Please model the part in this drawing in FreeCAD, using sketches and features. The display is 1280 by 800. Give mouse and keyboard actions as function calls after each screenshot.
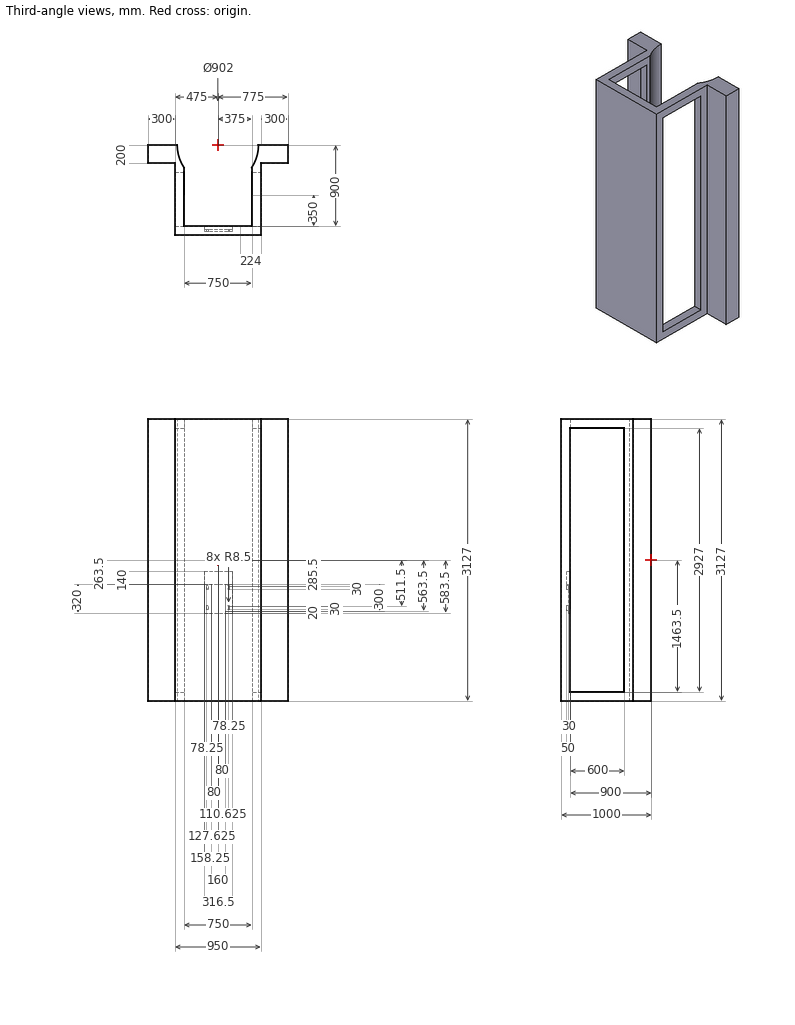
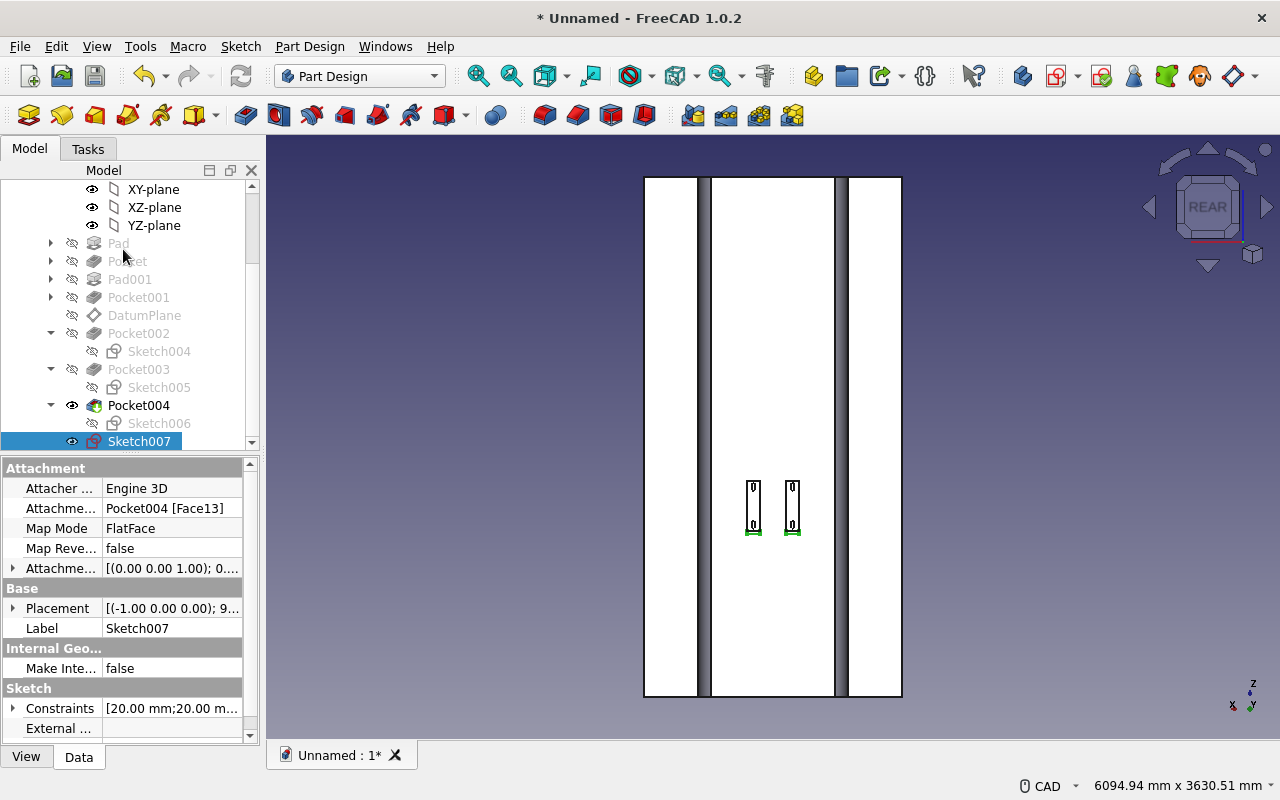
click(246, 116)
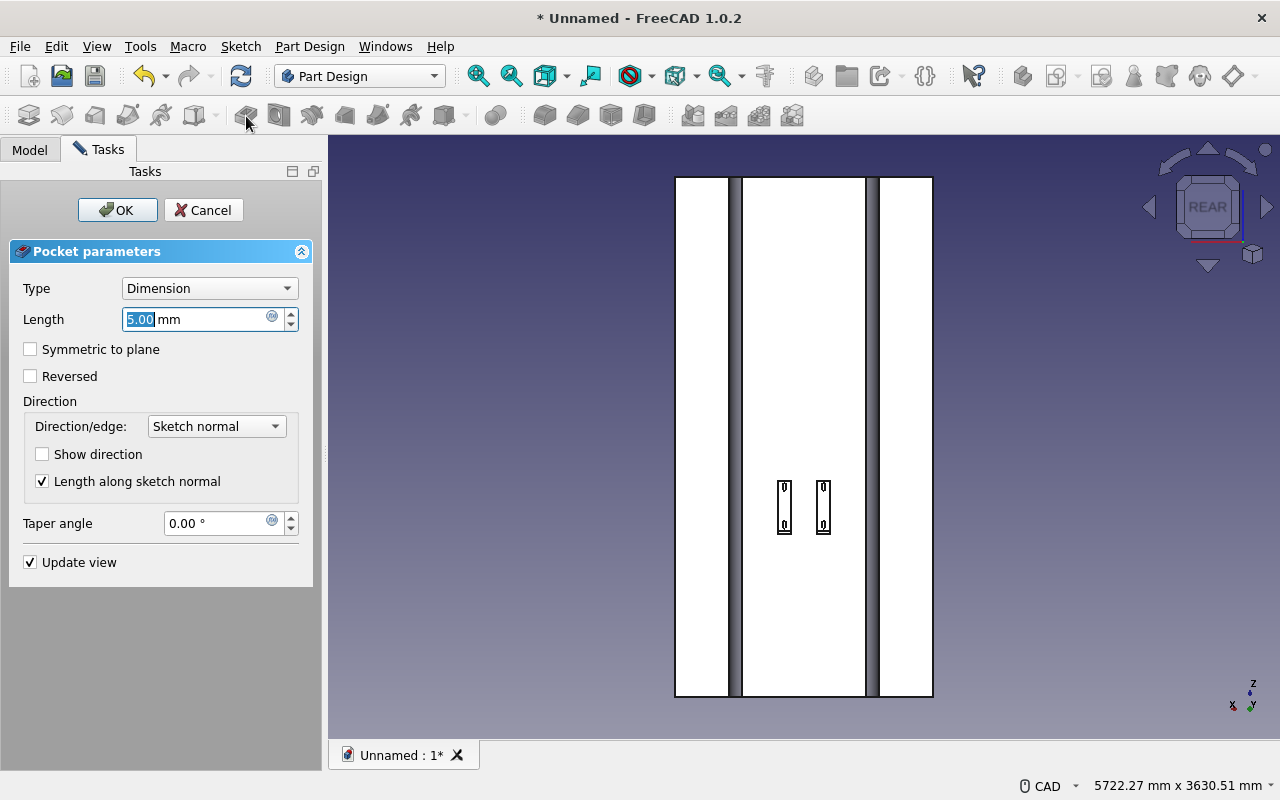
text(30)
key(Tab)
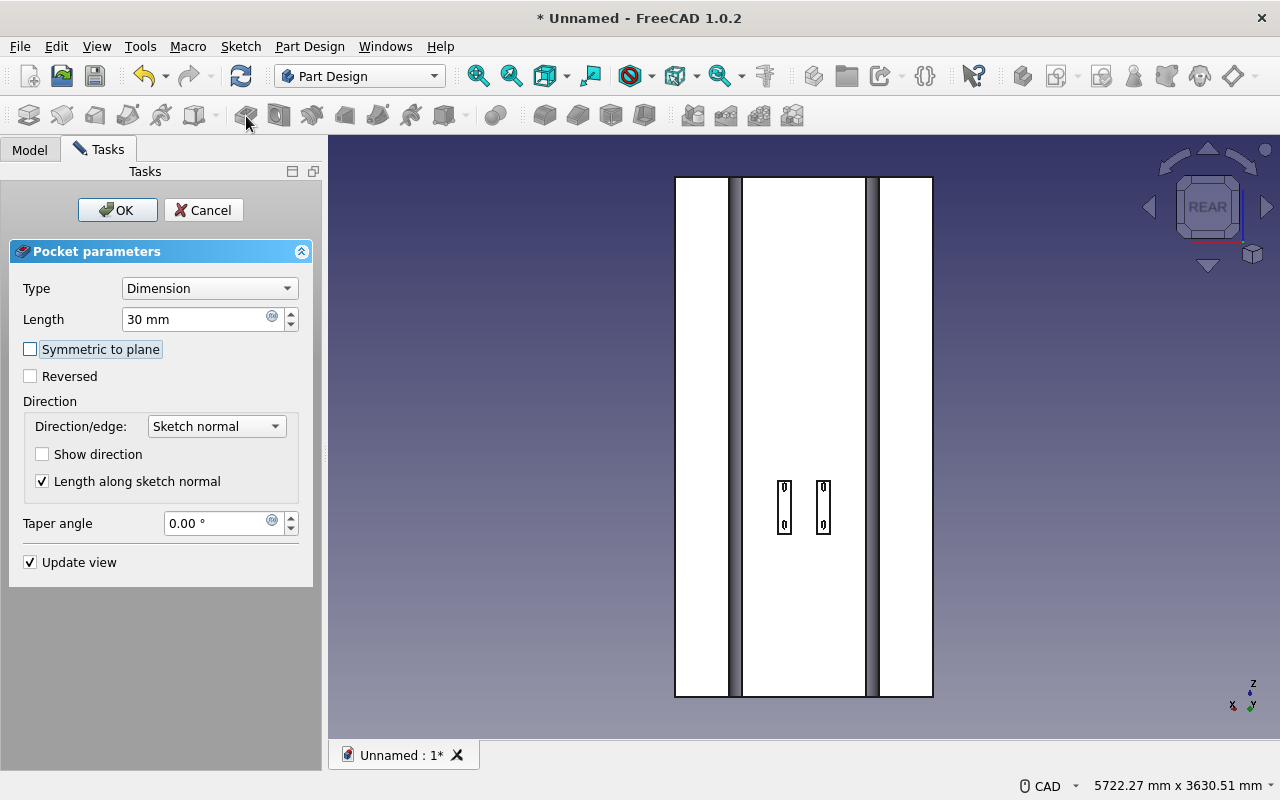
click(118, 210)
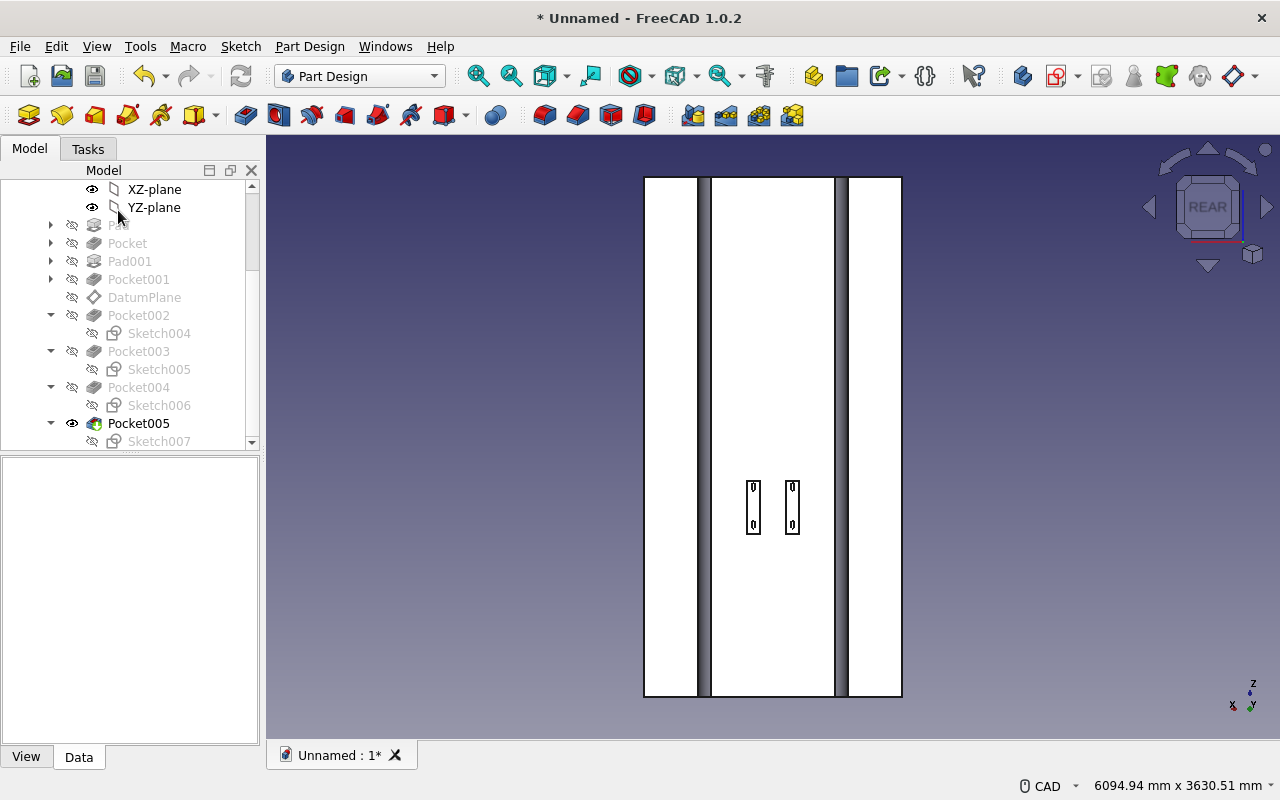
click(773, 287)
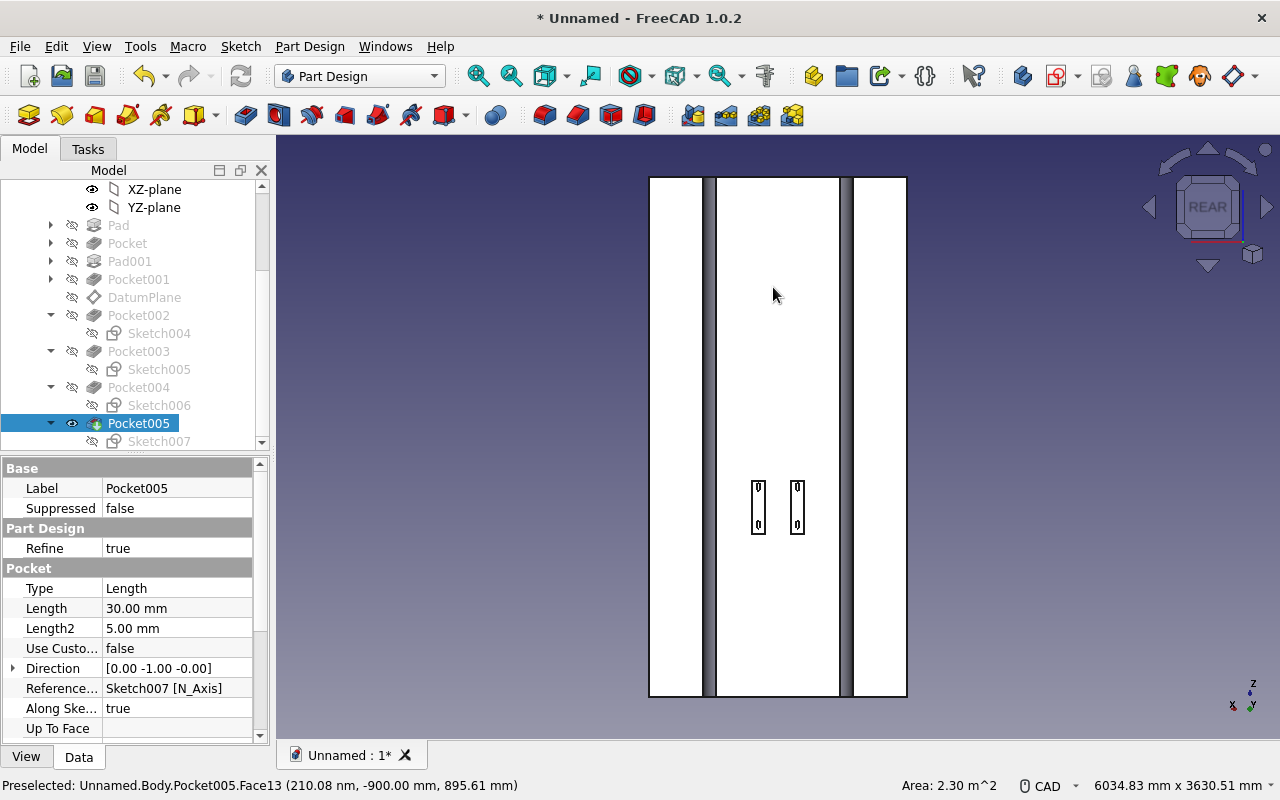
click(1056, 76)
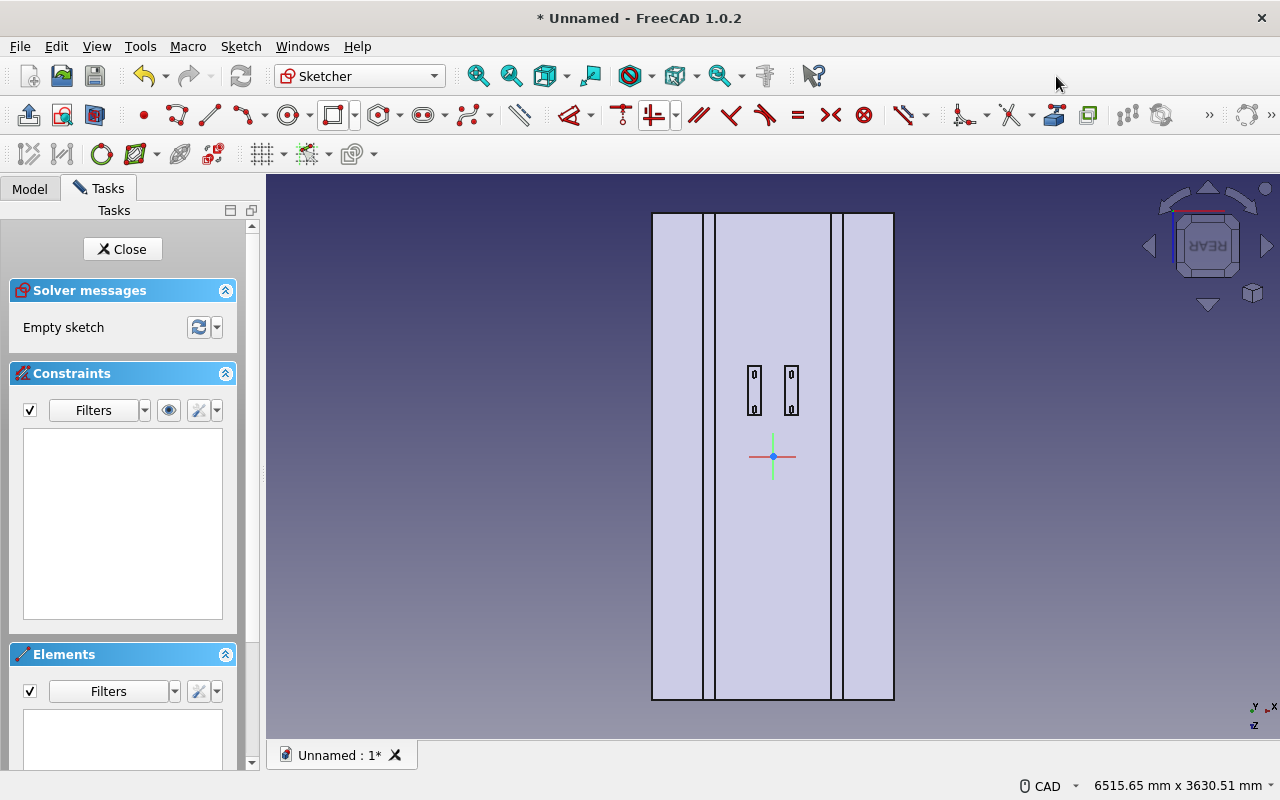
scroll(795, 396, up, 7)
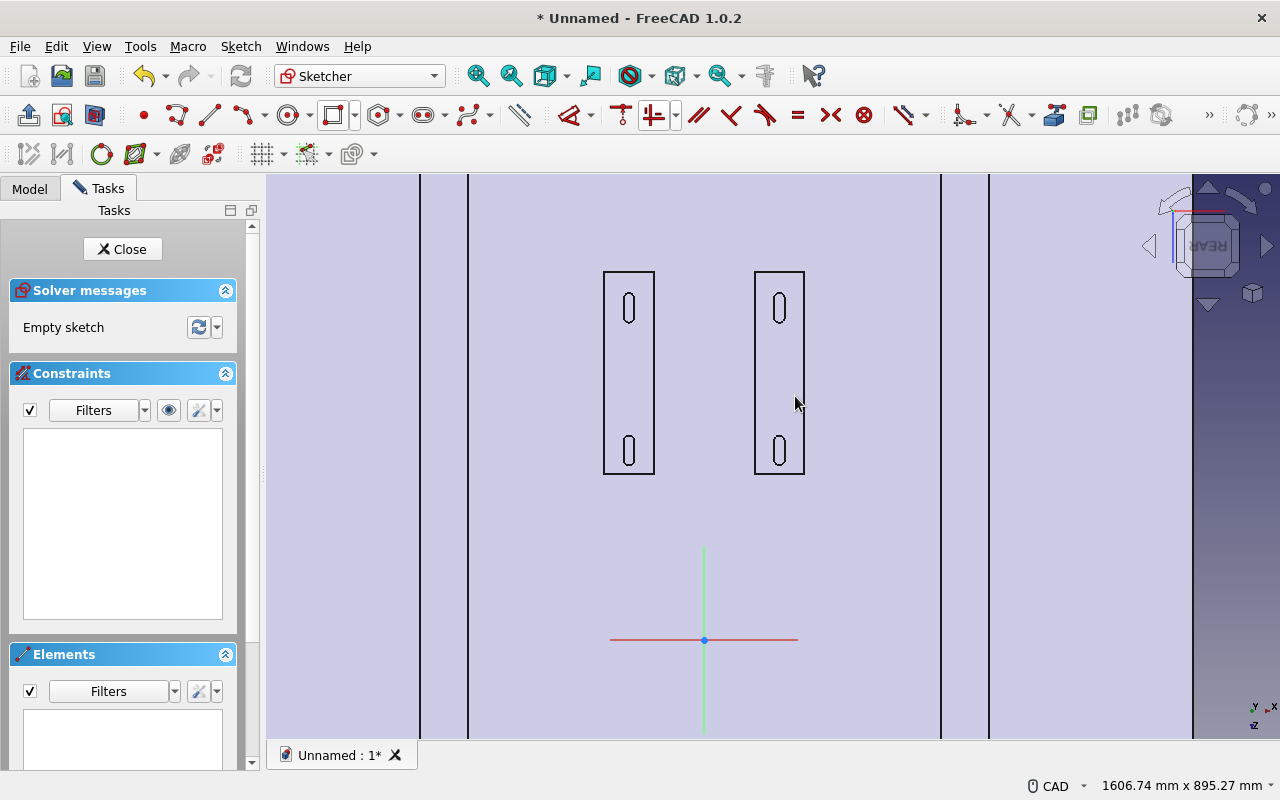
click(332, 116)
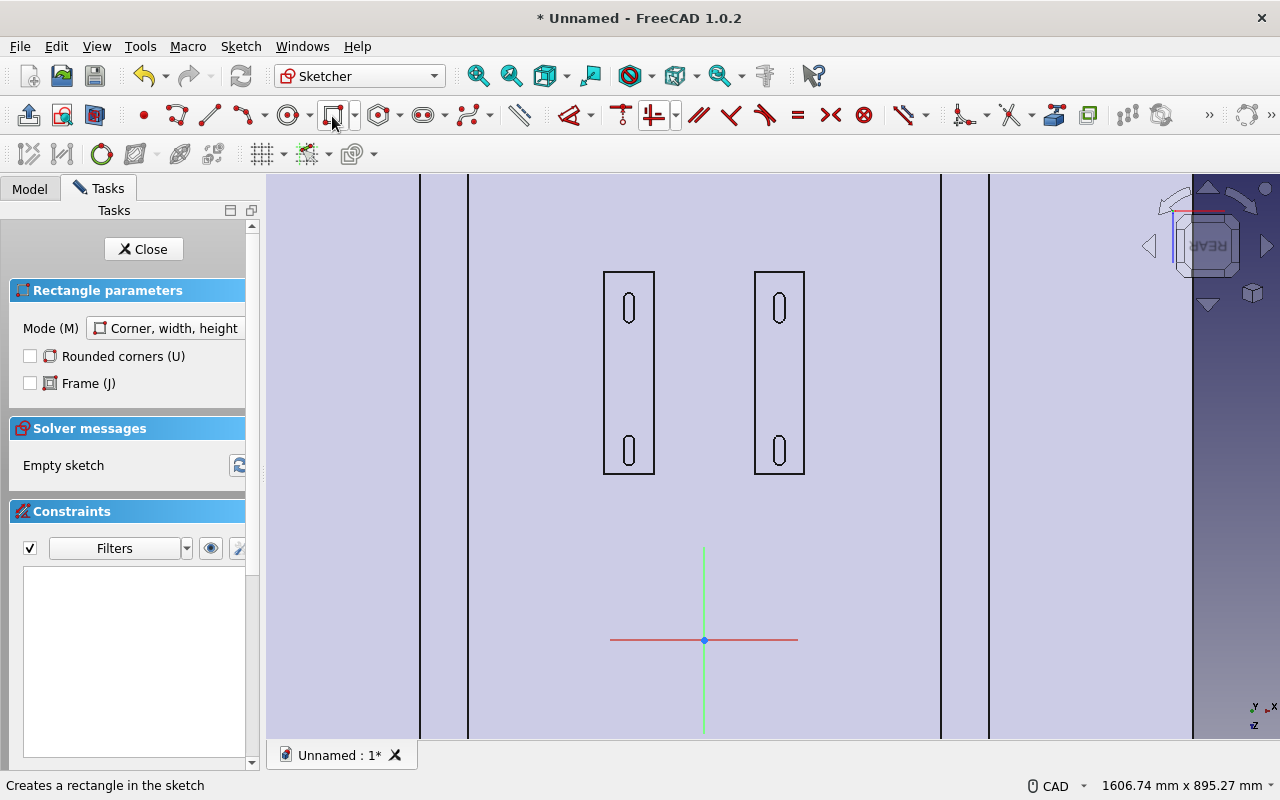
click(654, 272)
click(755, 474)
key(Escape)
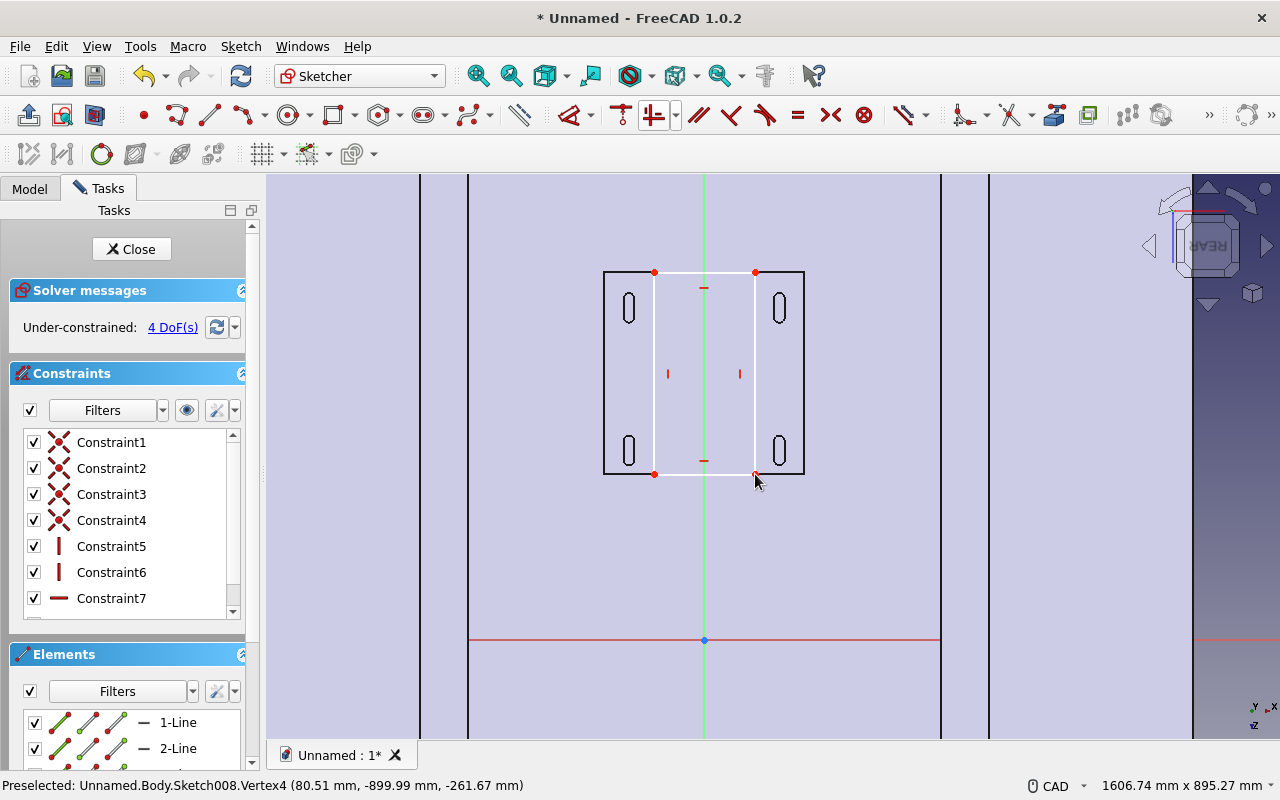
click(568, 116)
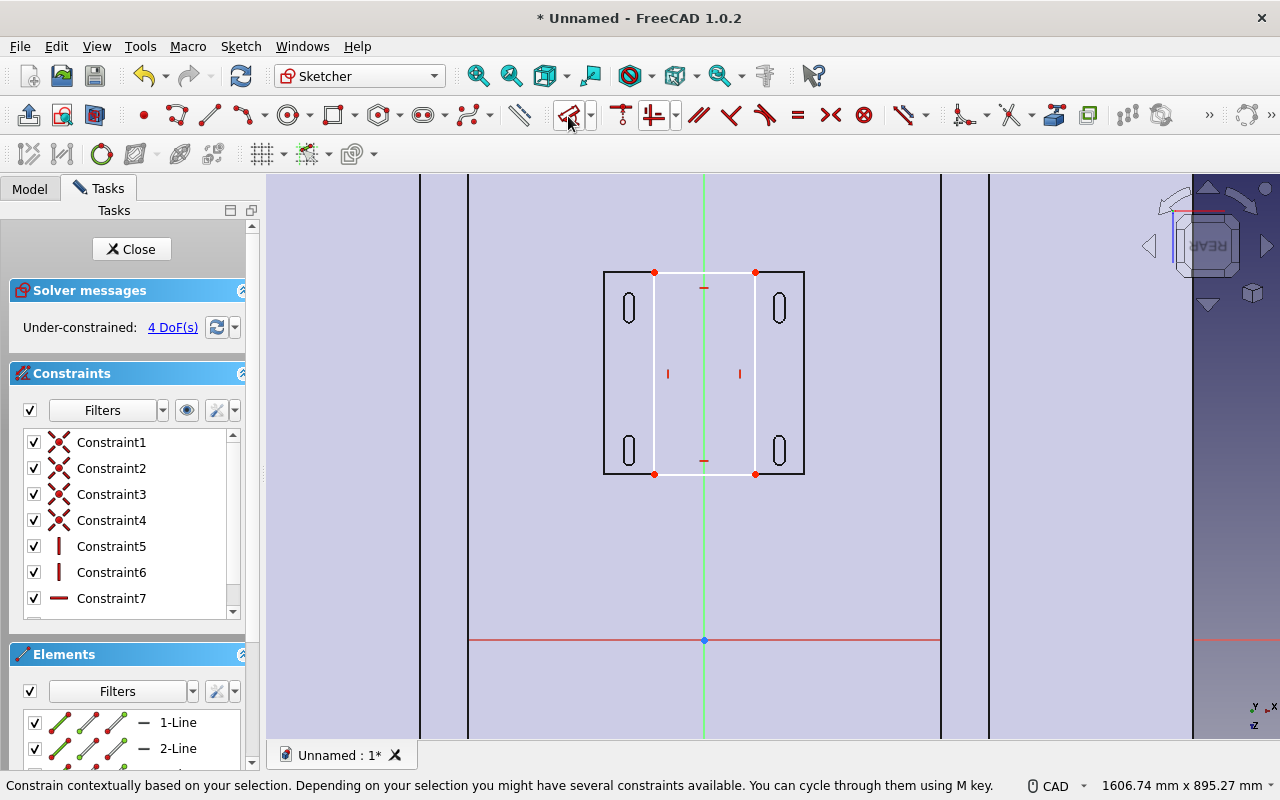
click(654, 334)
click(620, 374)